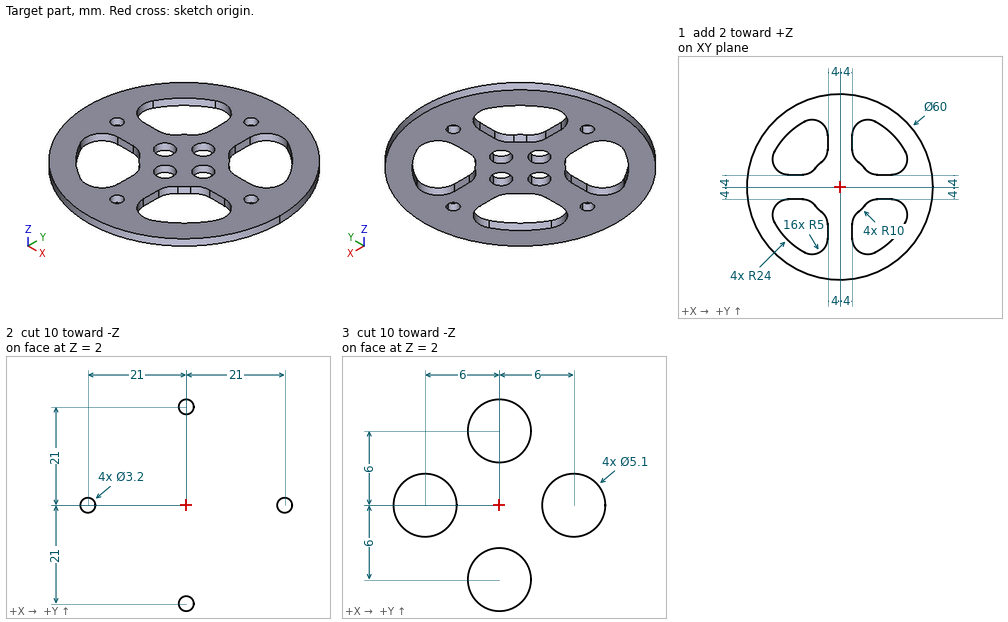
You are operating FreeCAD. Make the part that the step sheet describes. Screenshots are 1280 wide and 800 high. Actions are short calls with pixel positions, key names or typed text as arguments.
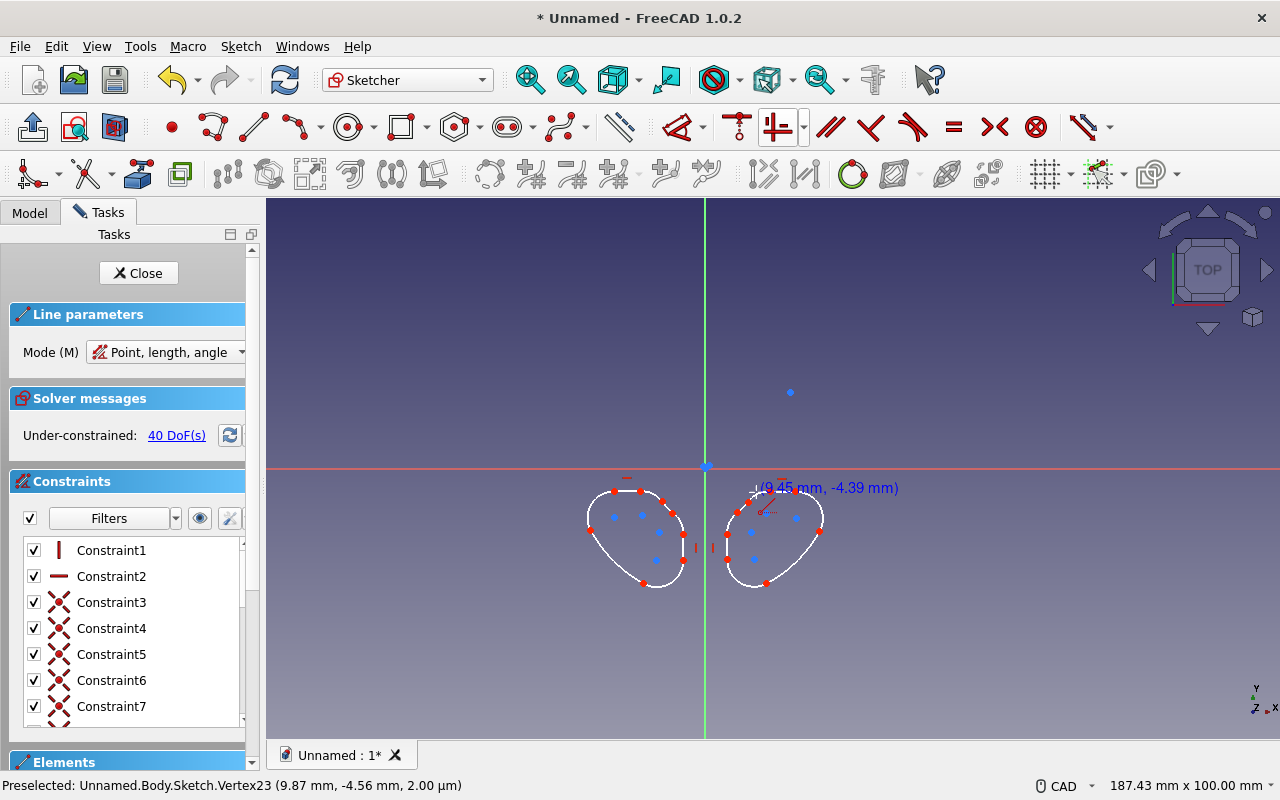
click(684, 378)
click(684, 404)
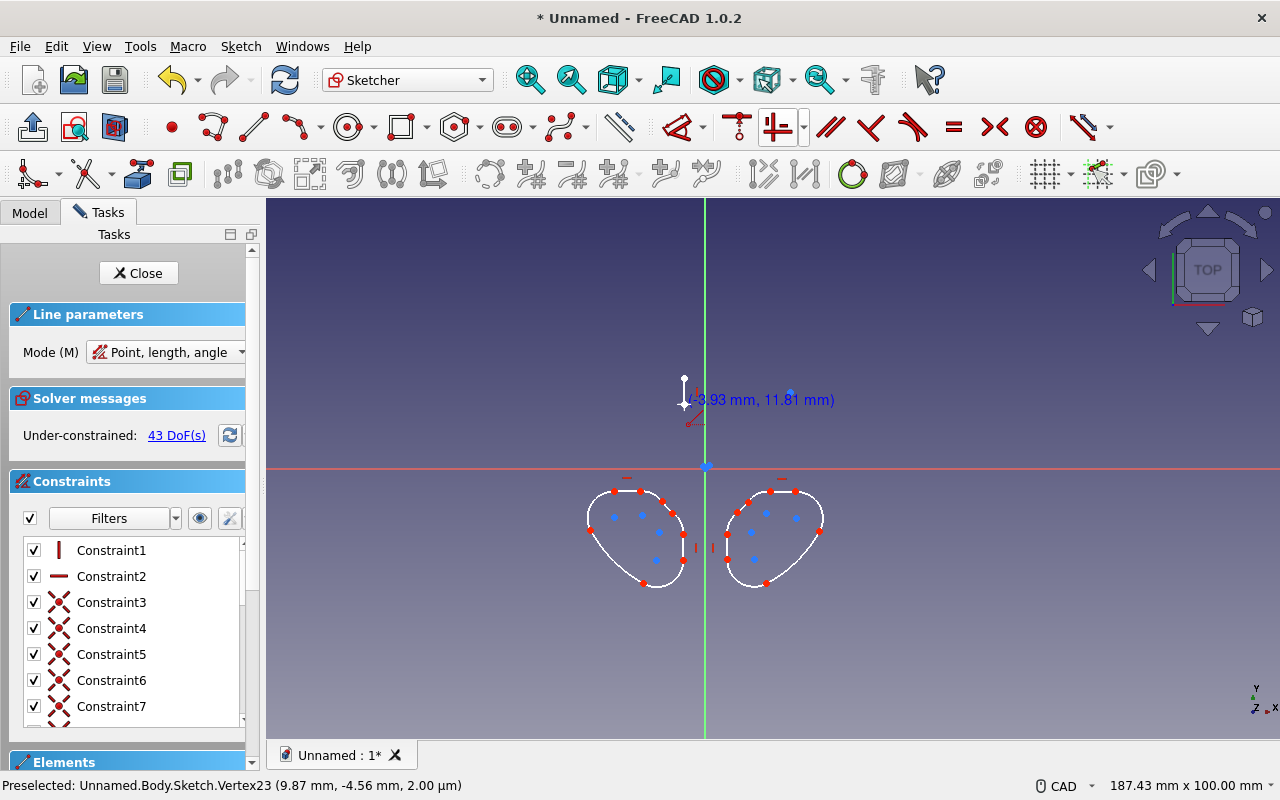
click(640, 447)
click(615, 447)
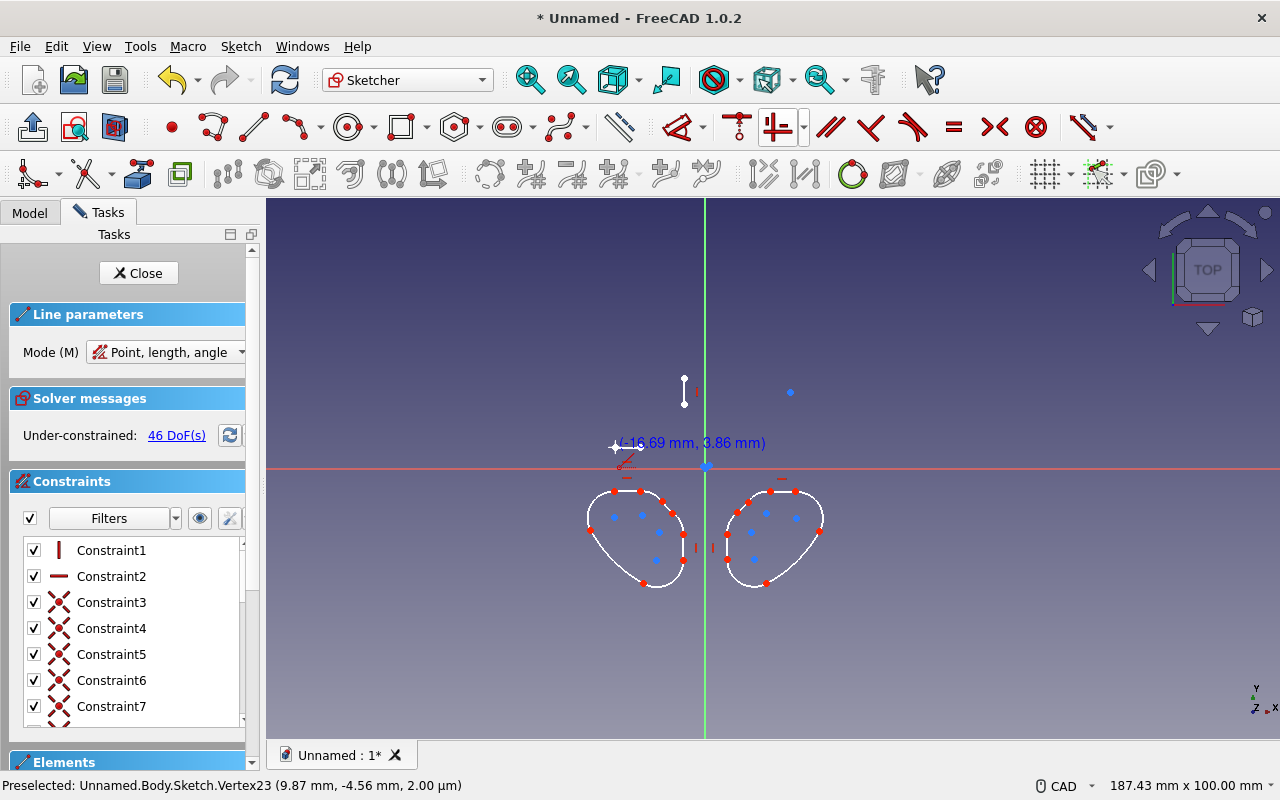
click(294, 128)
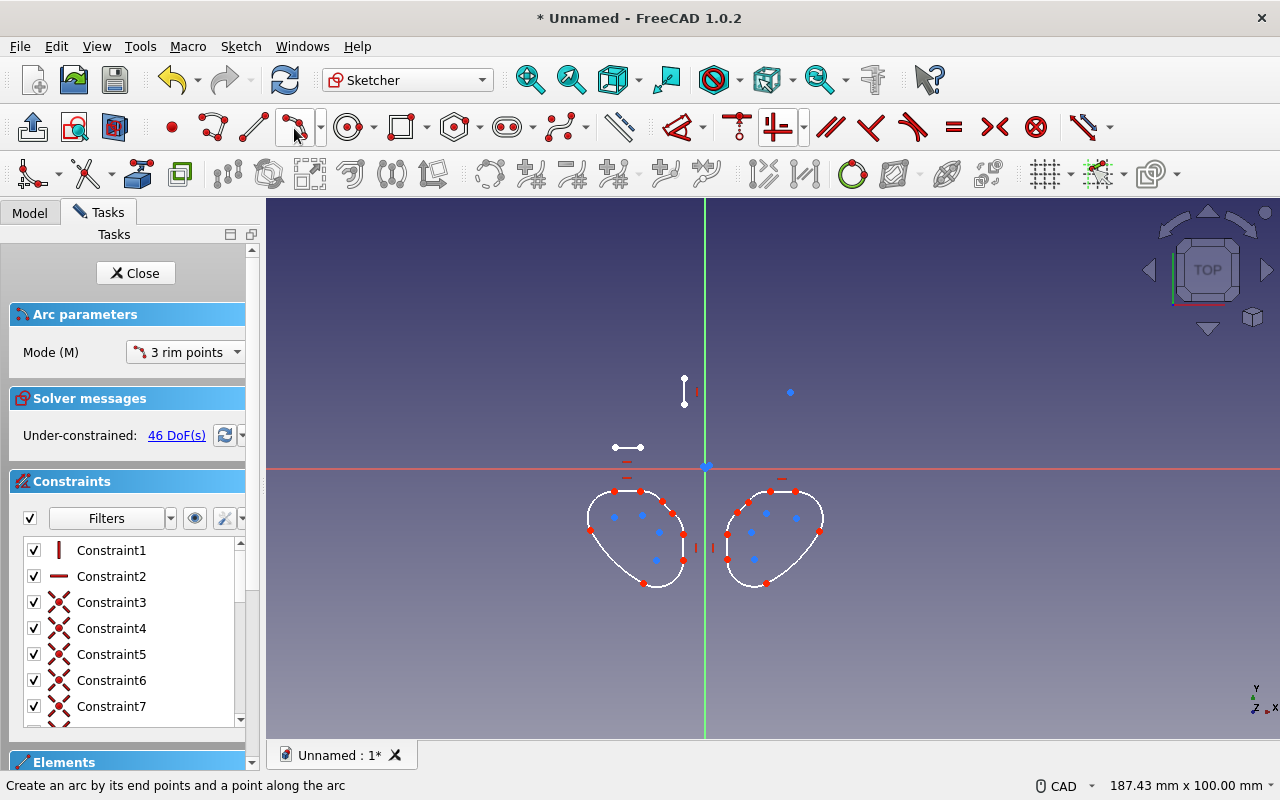
scroll(684, 404, up, 2)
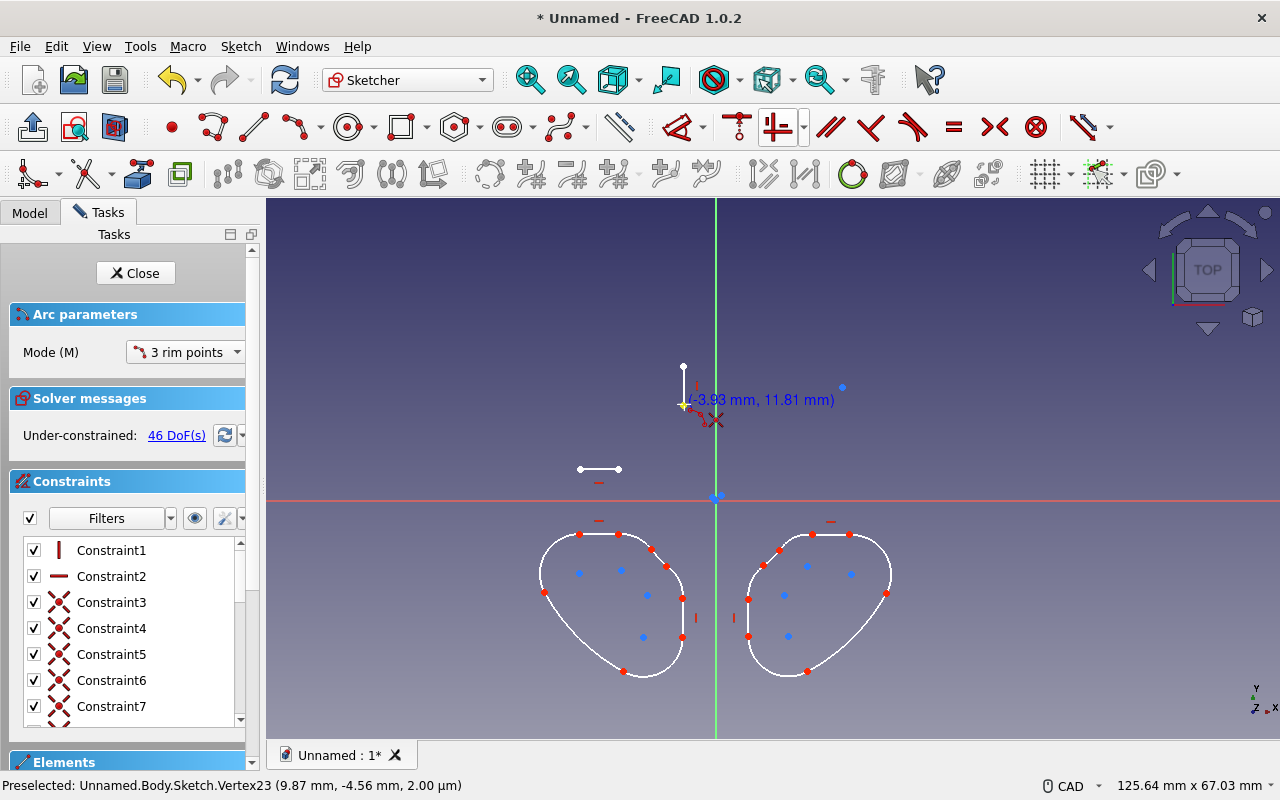
click(684, 405)
click(667, 436)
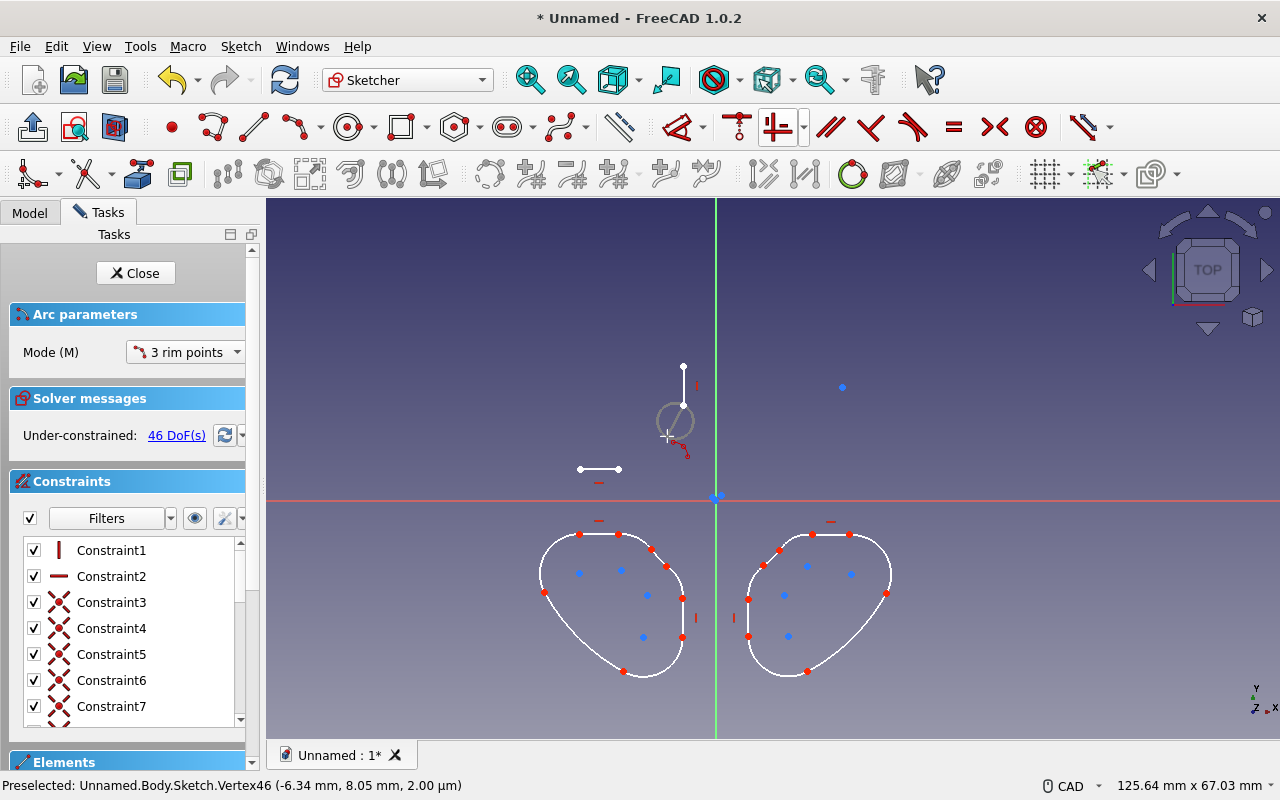
scroll(679, 422, up, 7)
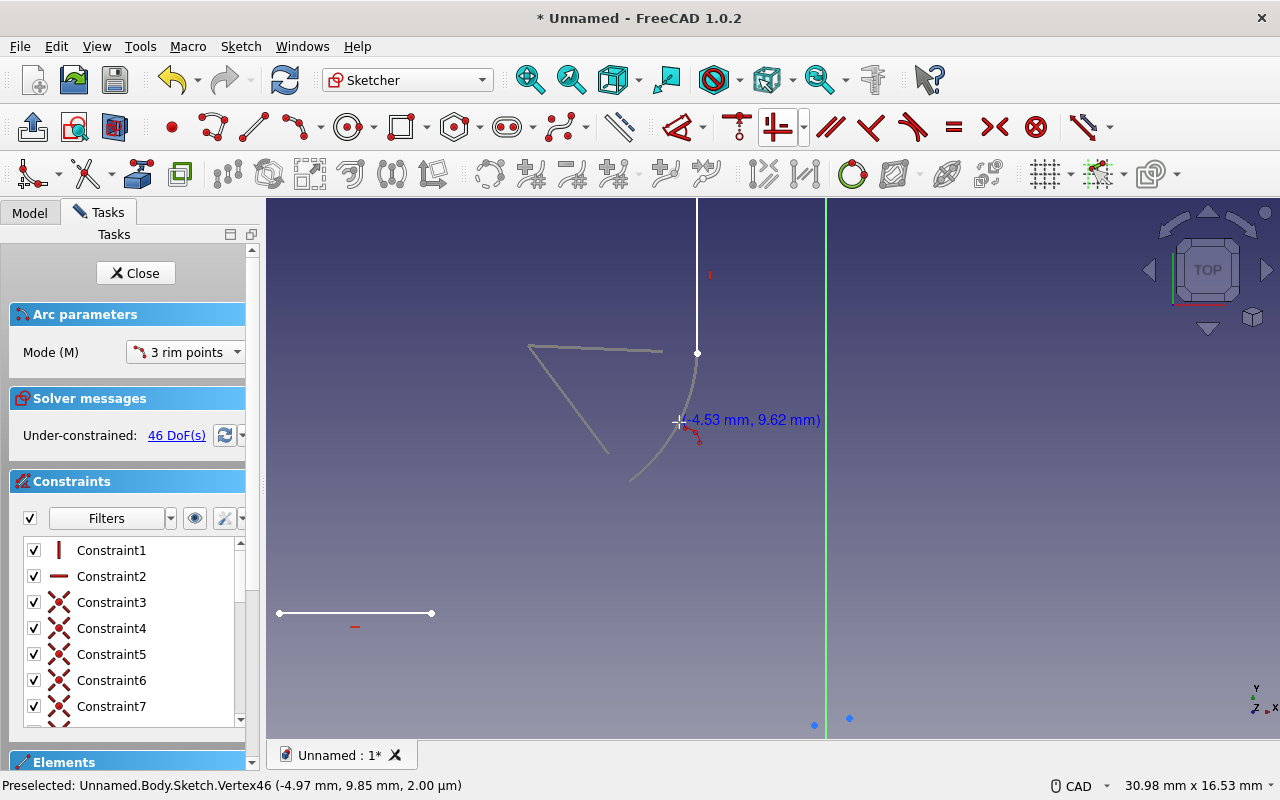
click(678, 420)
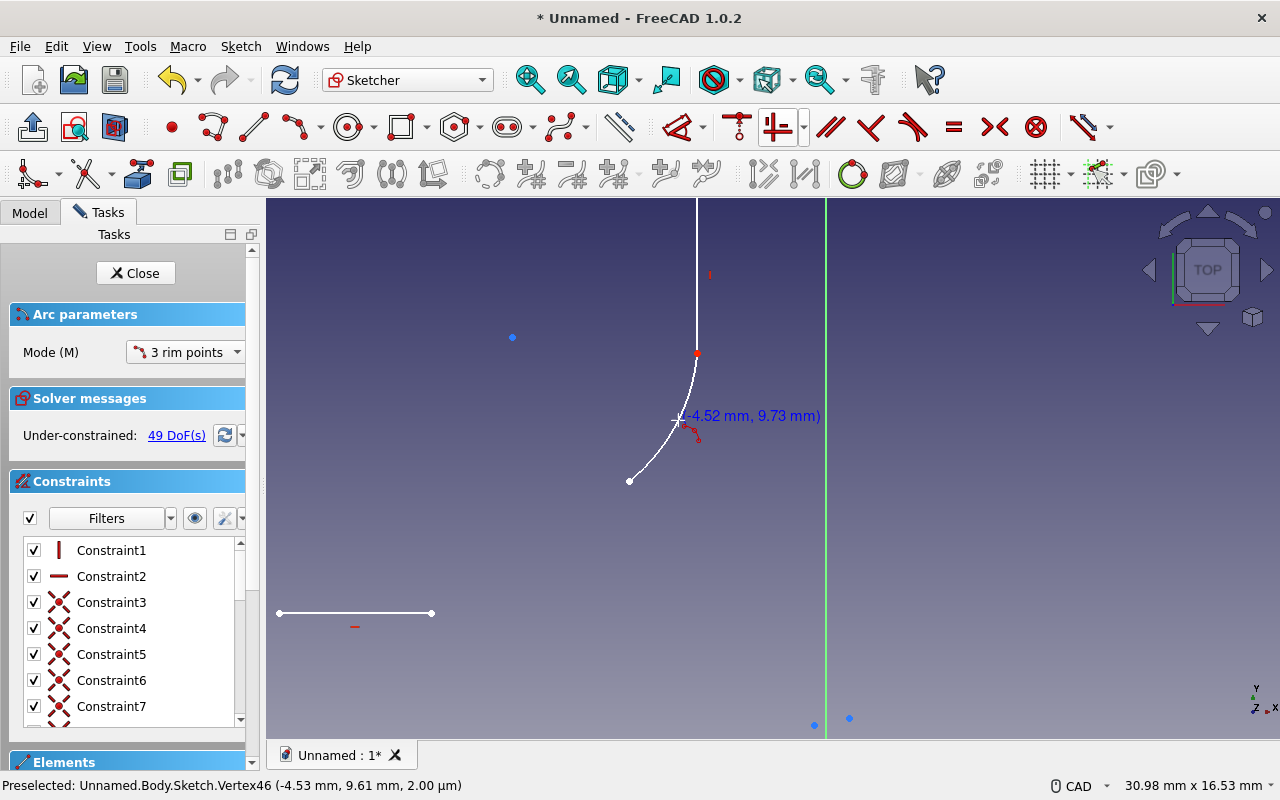
scroll(680, 415, down, 9)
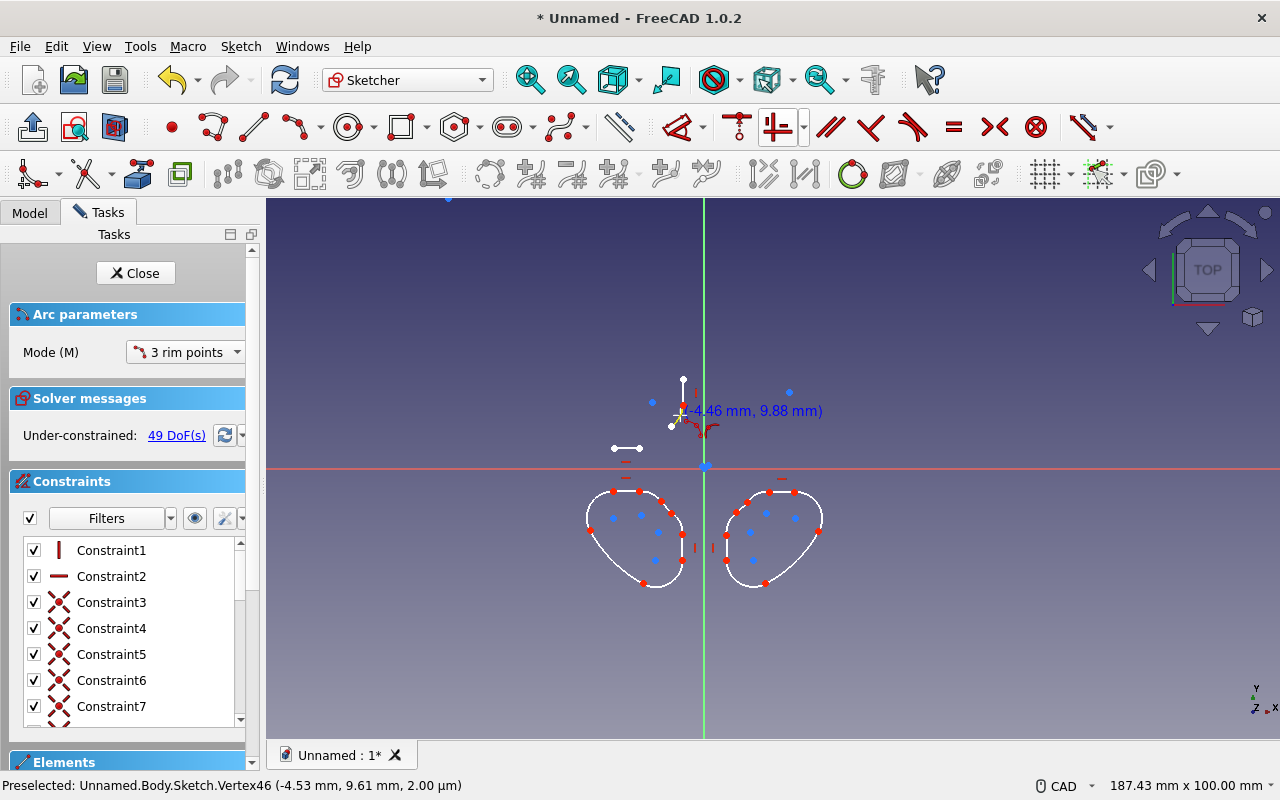
click(672, 426)
click(661, 437)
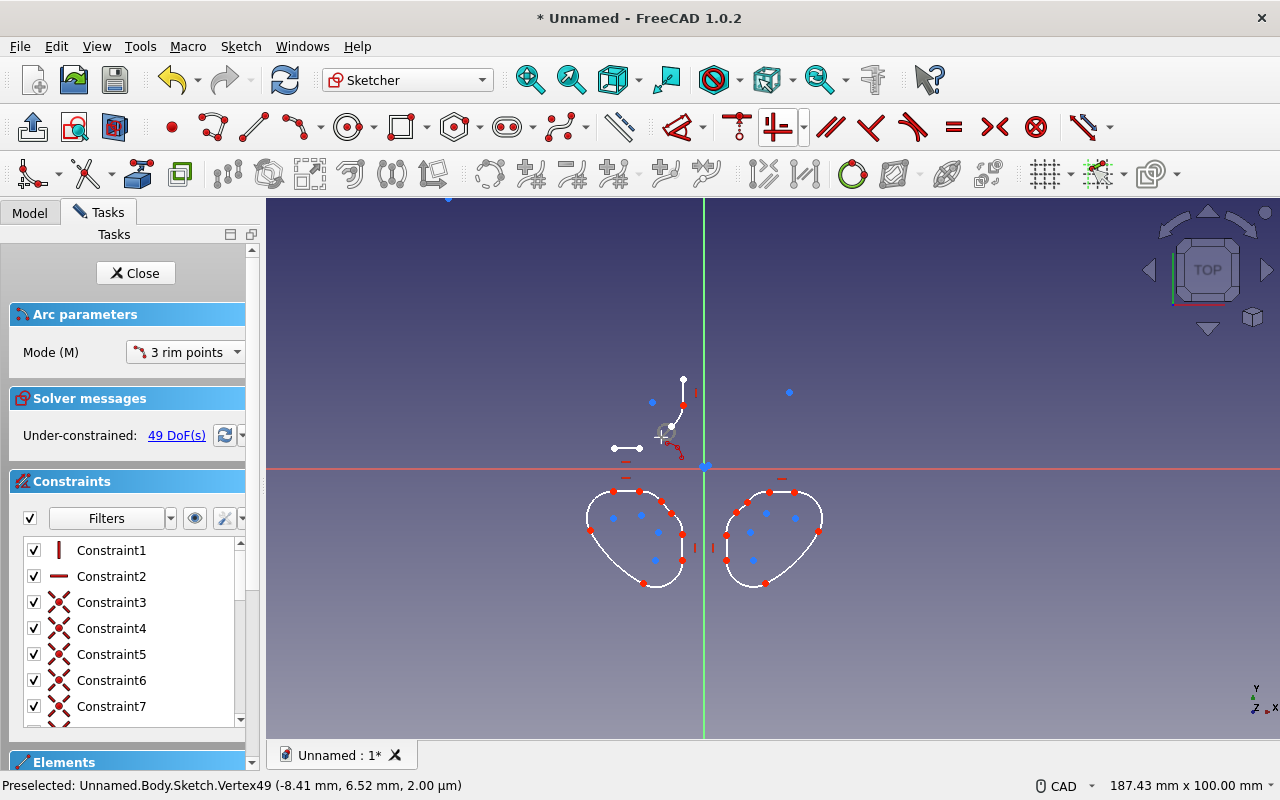
scroll(666, 431, up, 17)